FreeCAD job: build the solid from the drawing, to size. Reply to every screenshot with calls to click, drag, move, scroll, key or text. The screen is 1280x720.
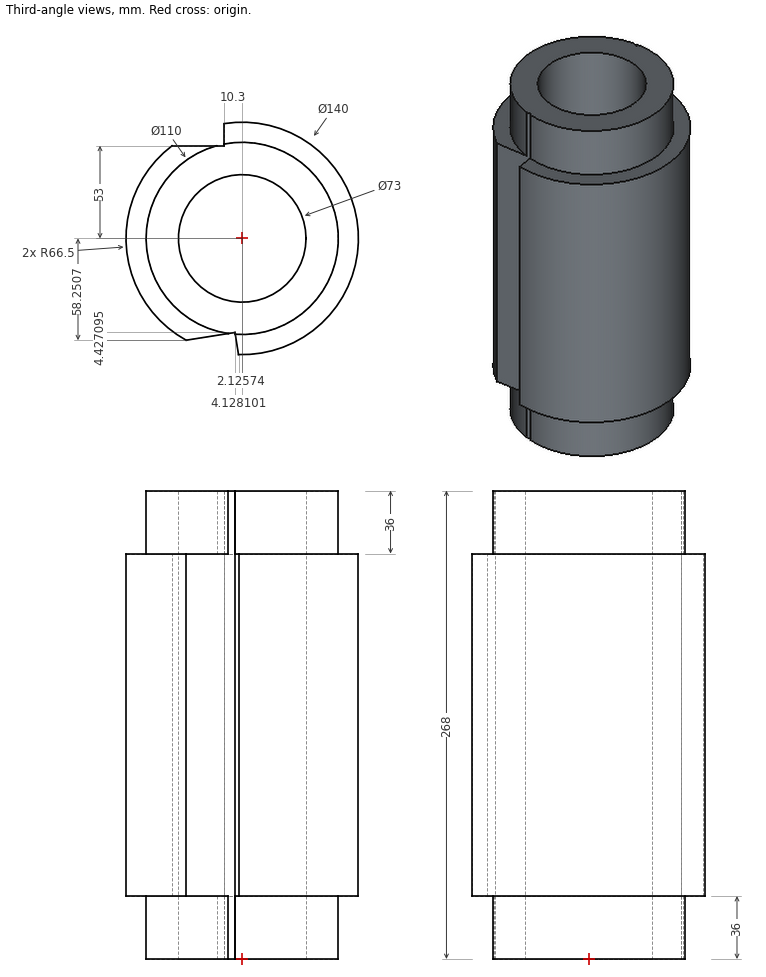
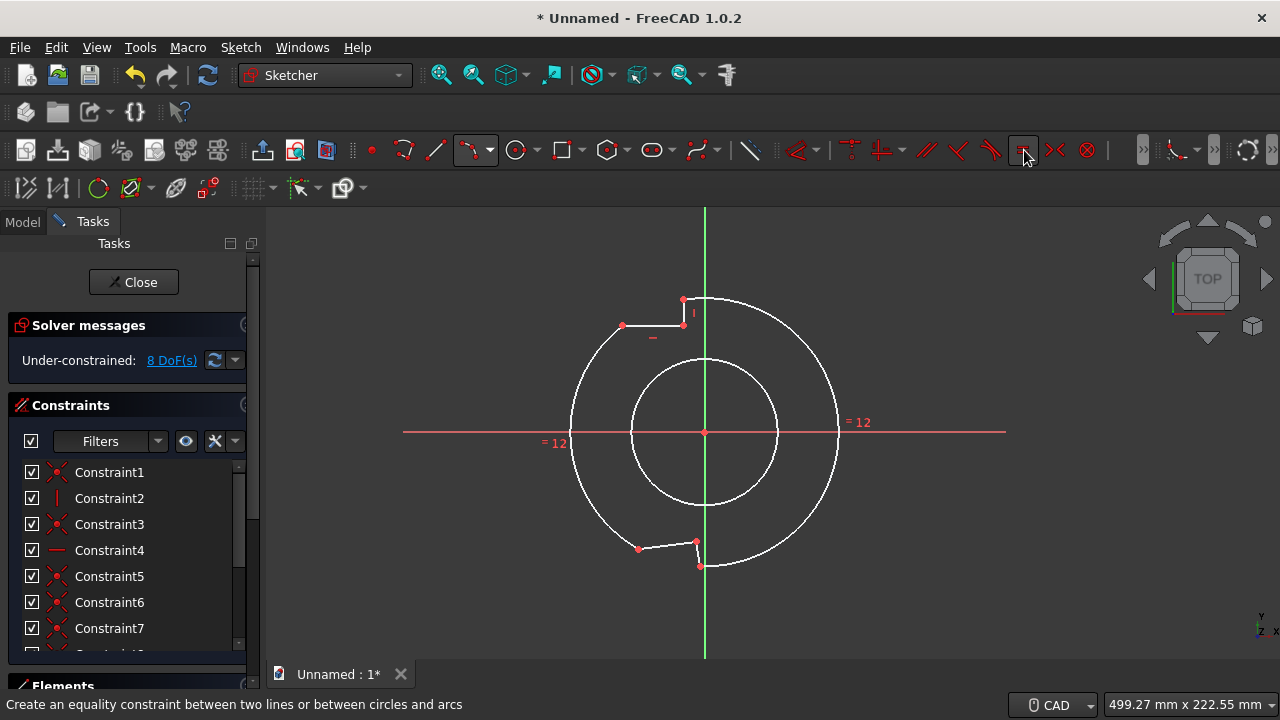
click(796, 150)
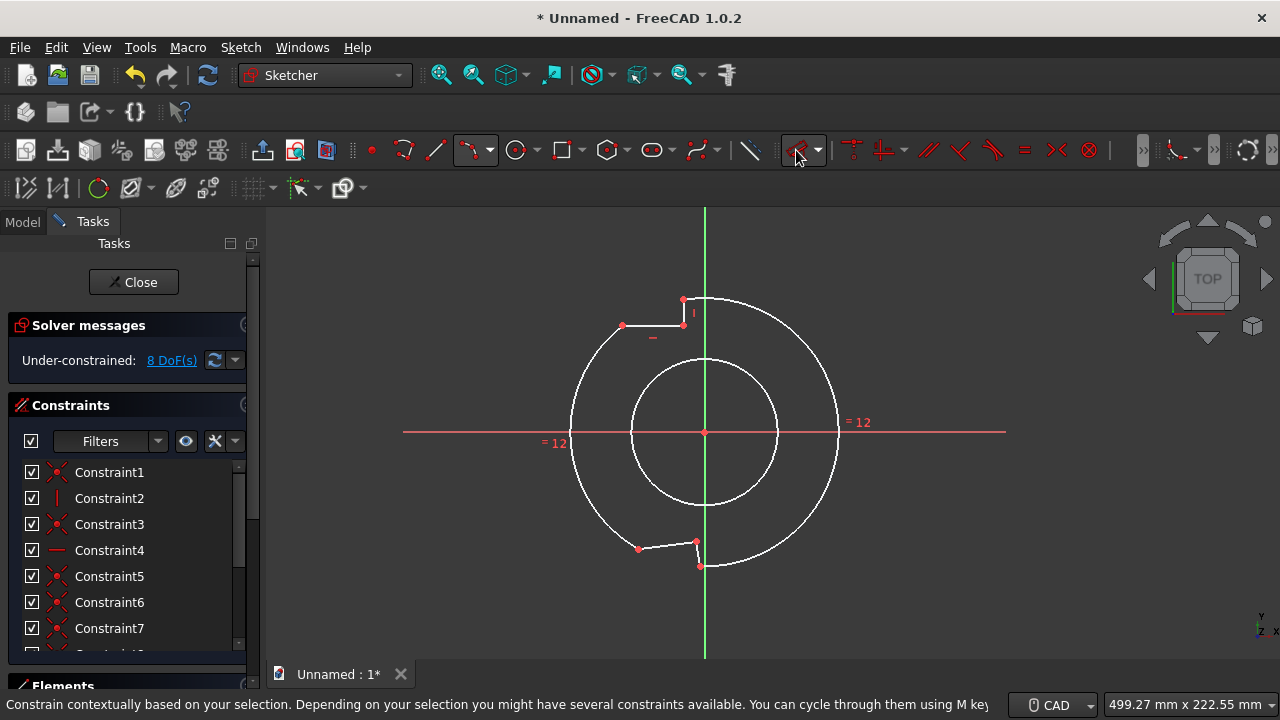
click(815, 508)
click(841, 526)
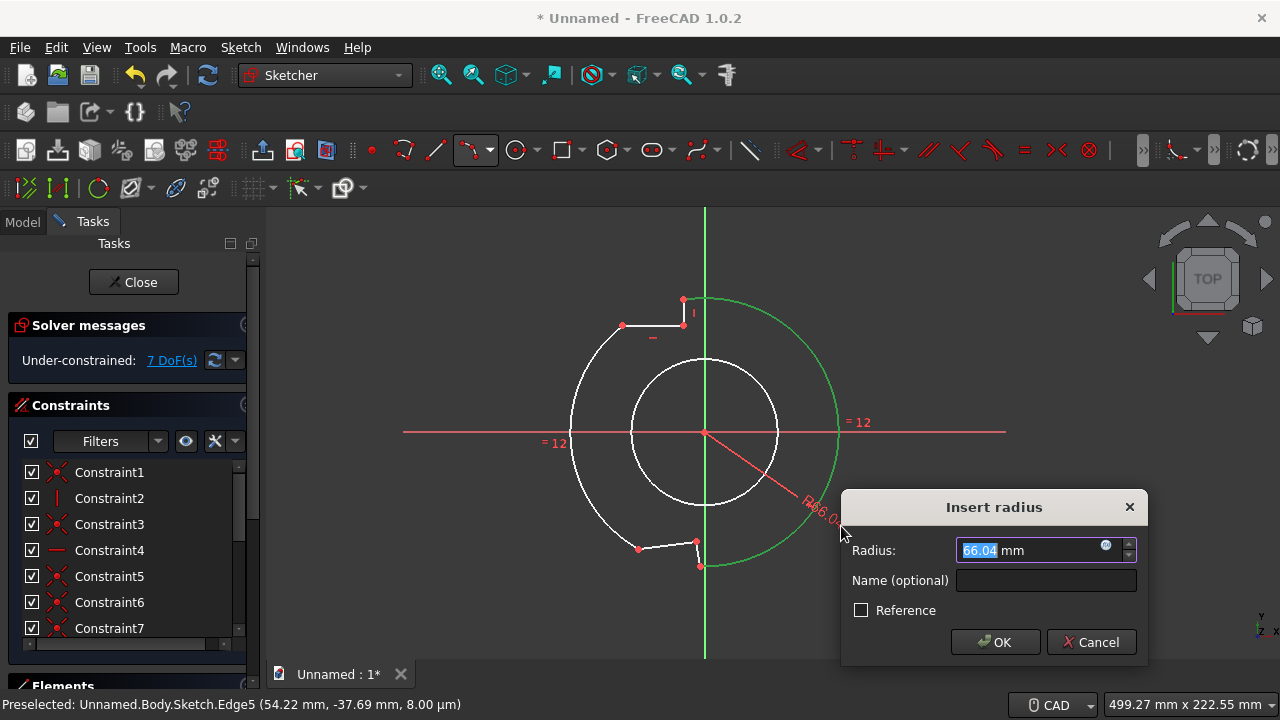
text(66.5)
key(Return)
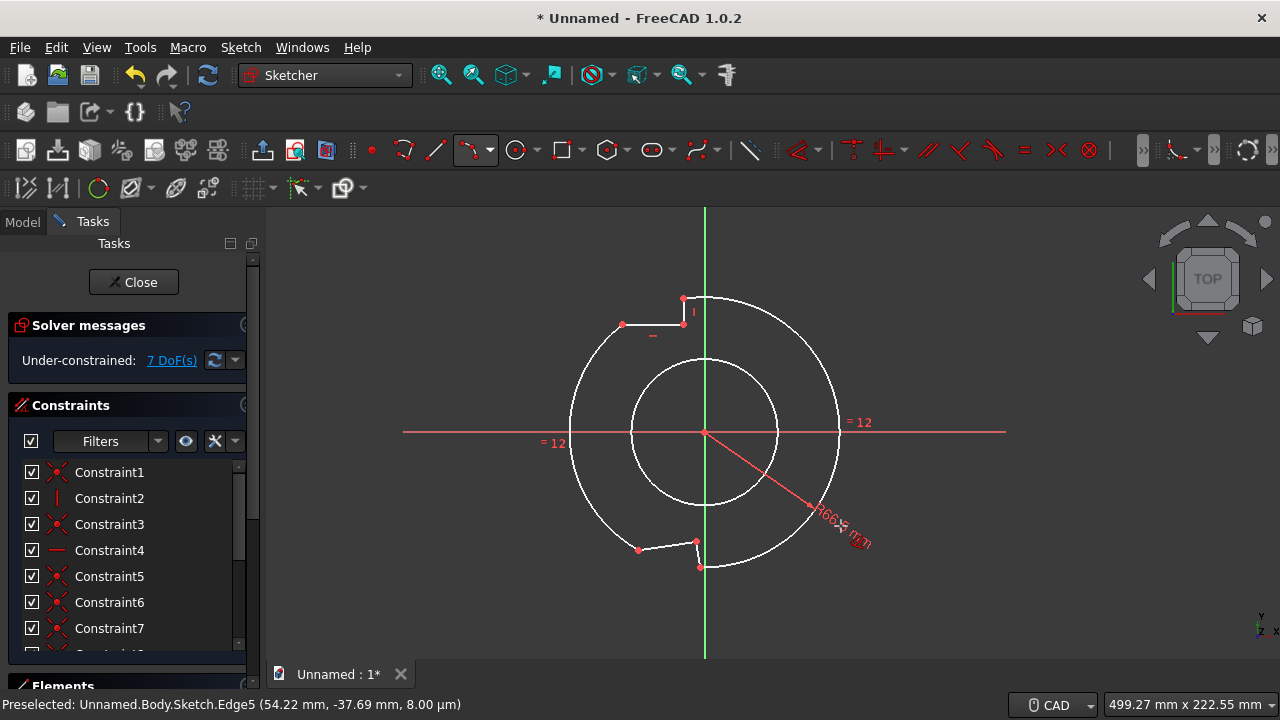
click(756, 380)
click(778, 357)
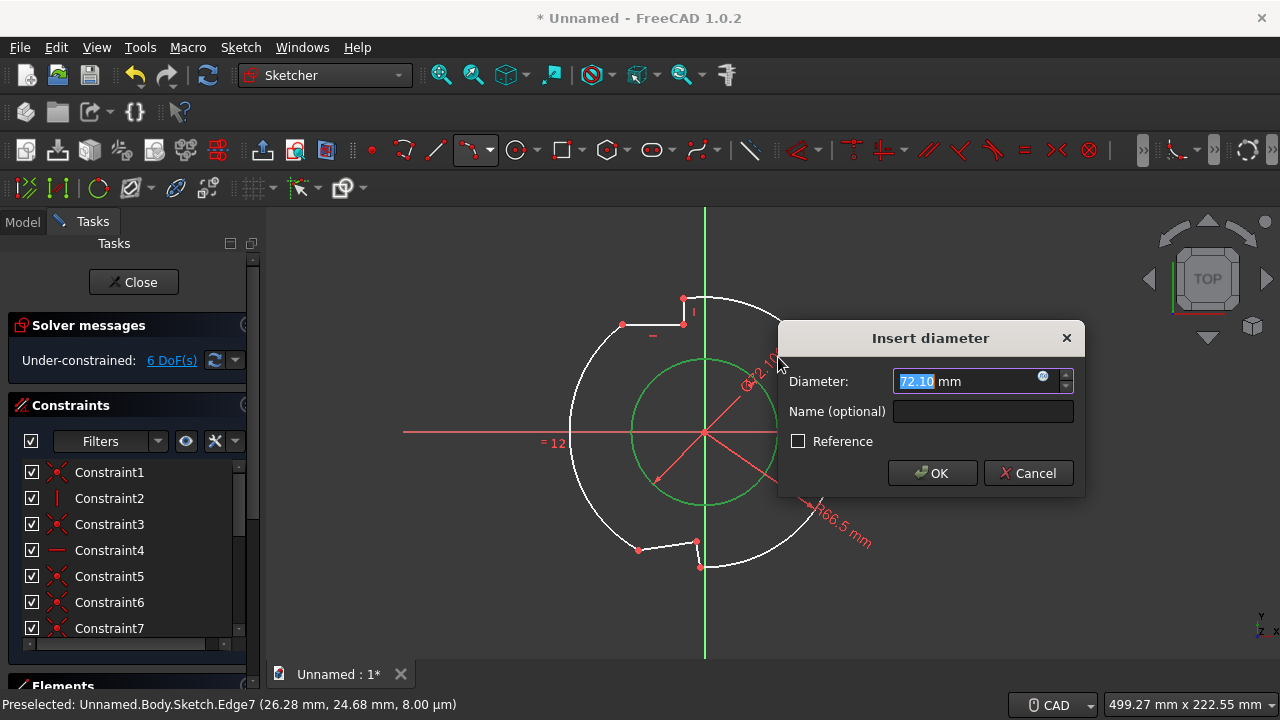
text(73)
key(Return)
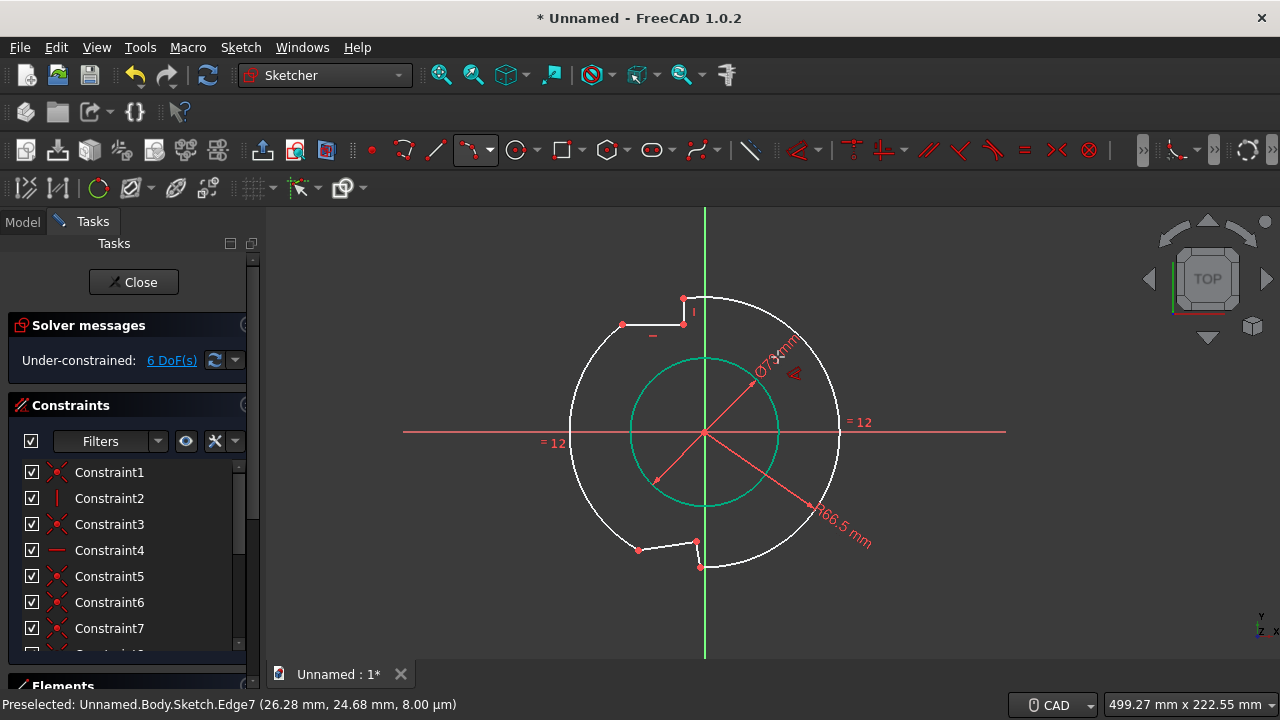
click(684, 325)
click(650, 354)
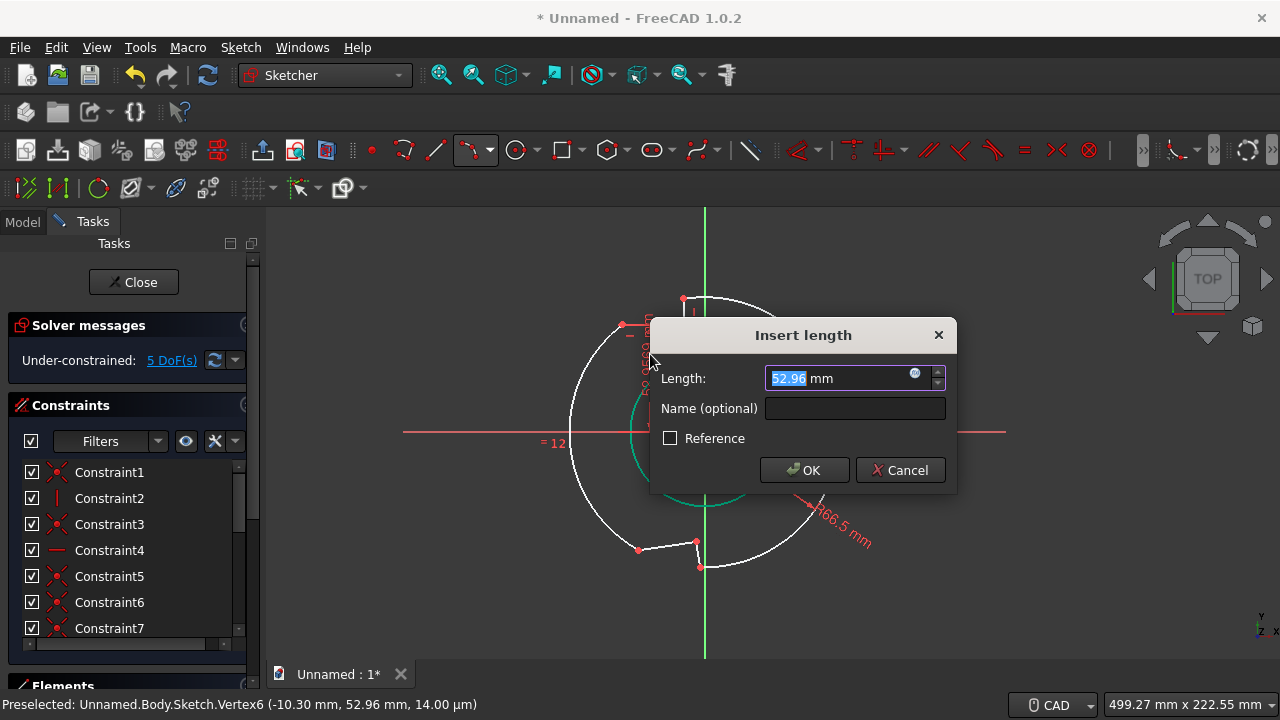
text(53)
key(Return)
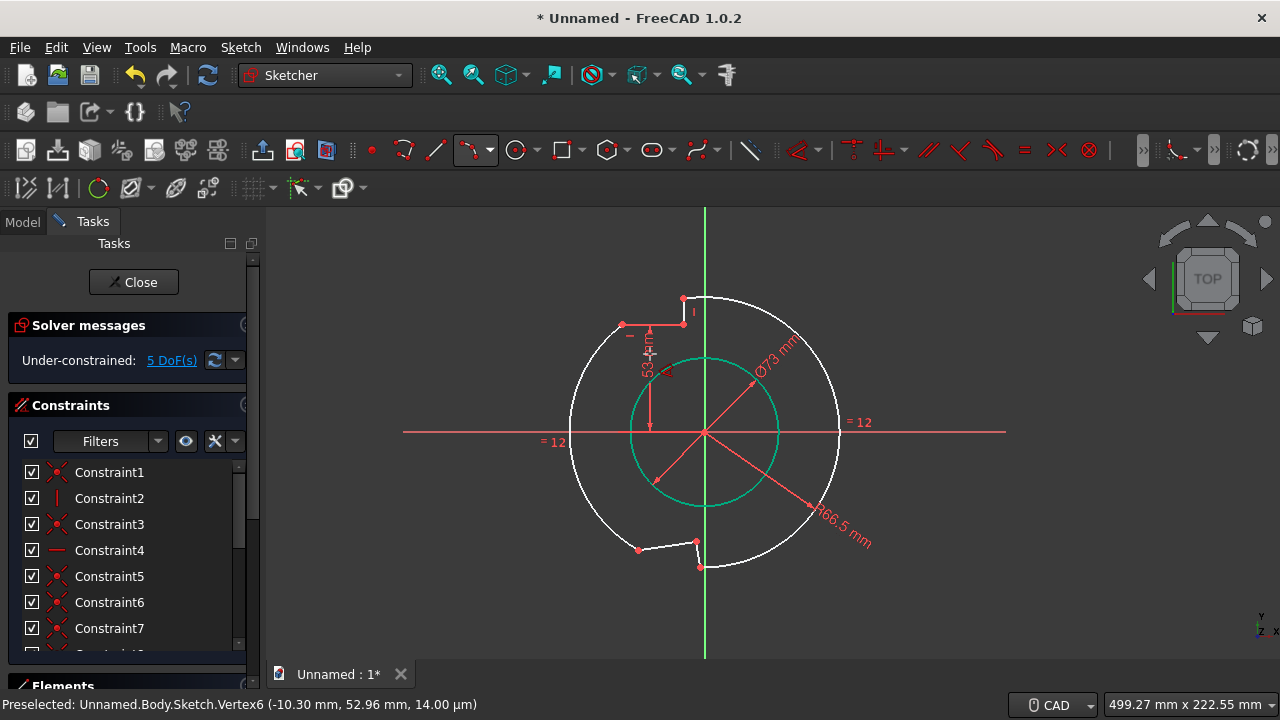
scroll(684, 299, up, 4)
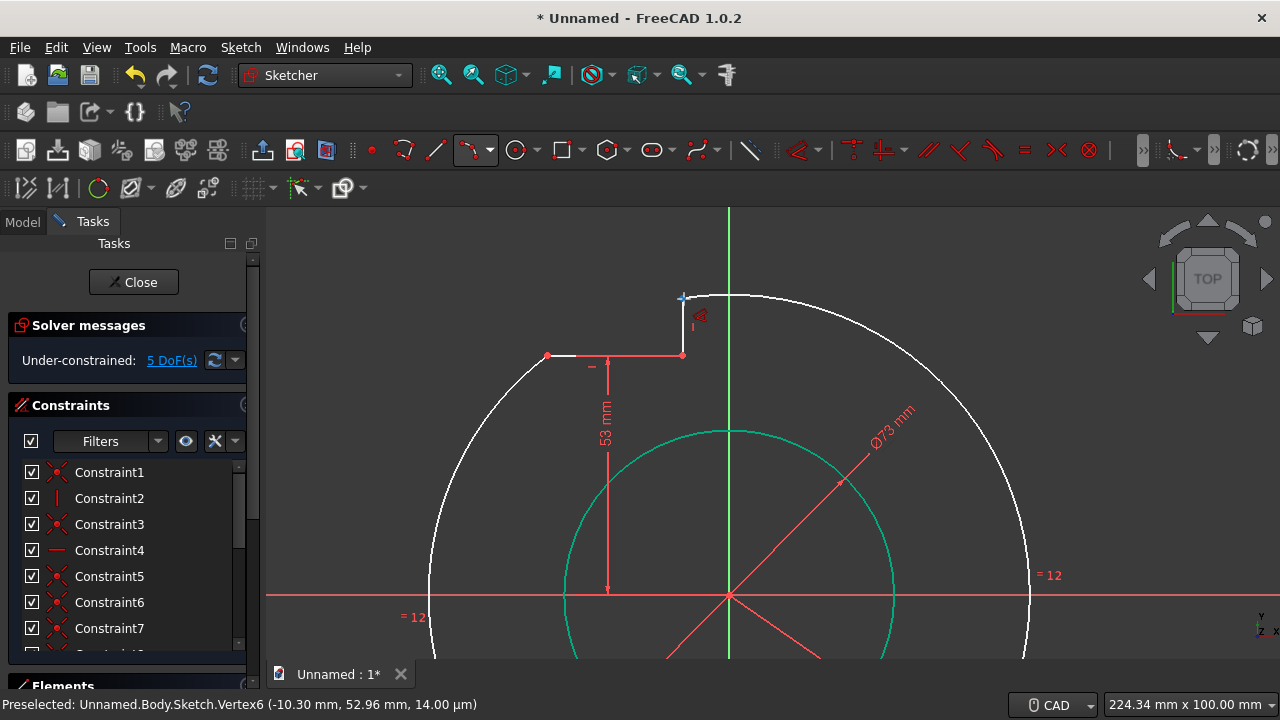
click(683, 298)
click(706, 264)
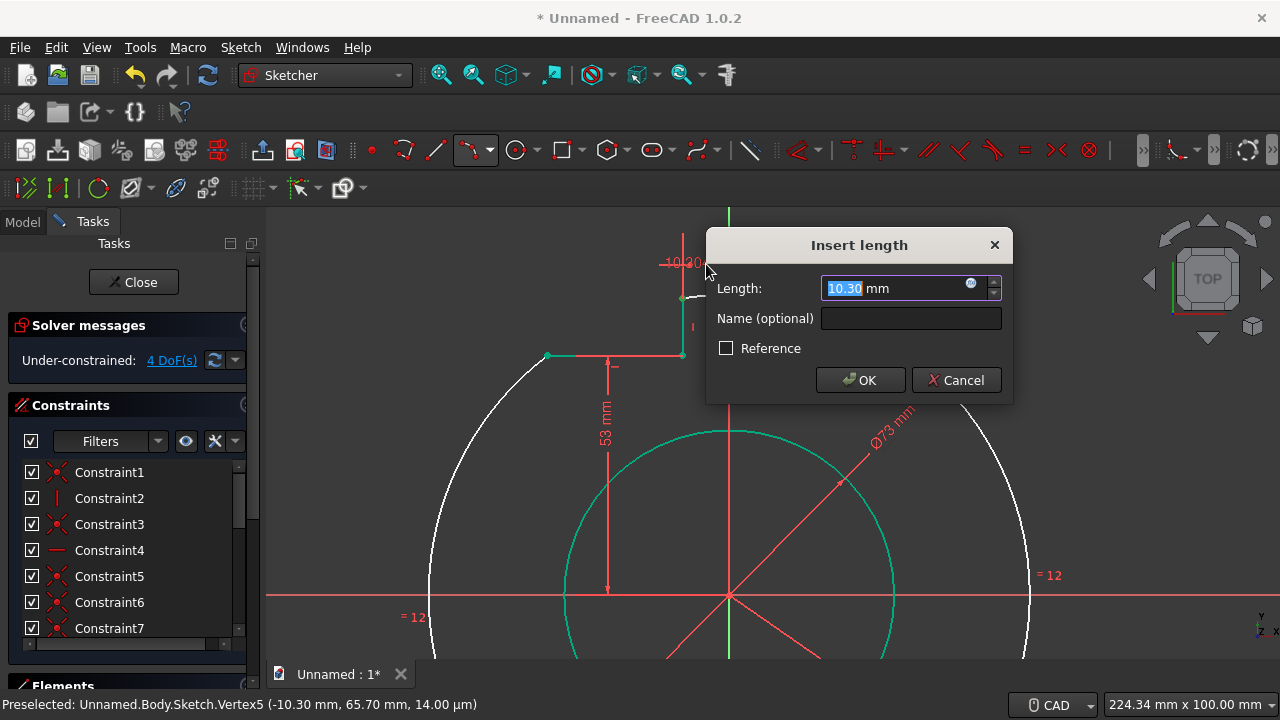
text(10.3)
key(Return)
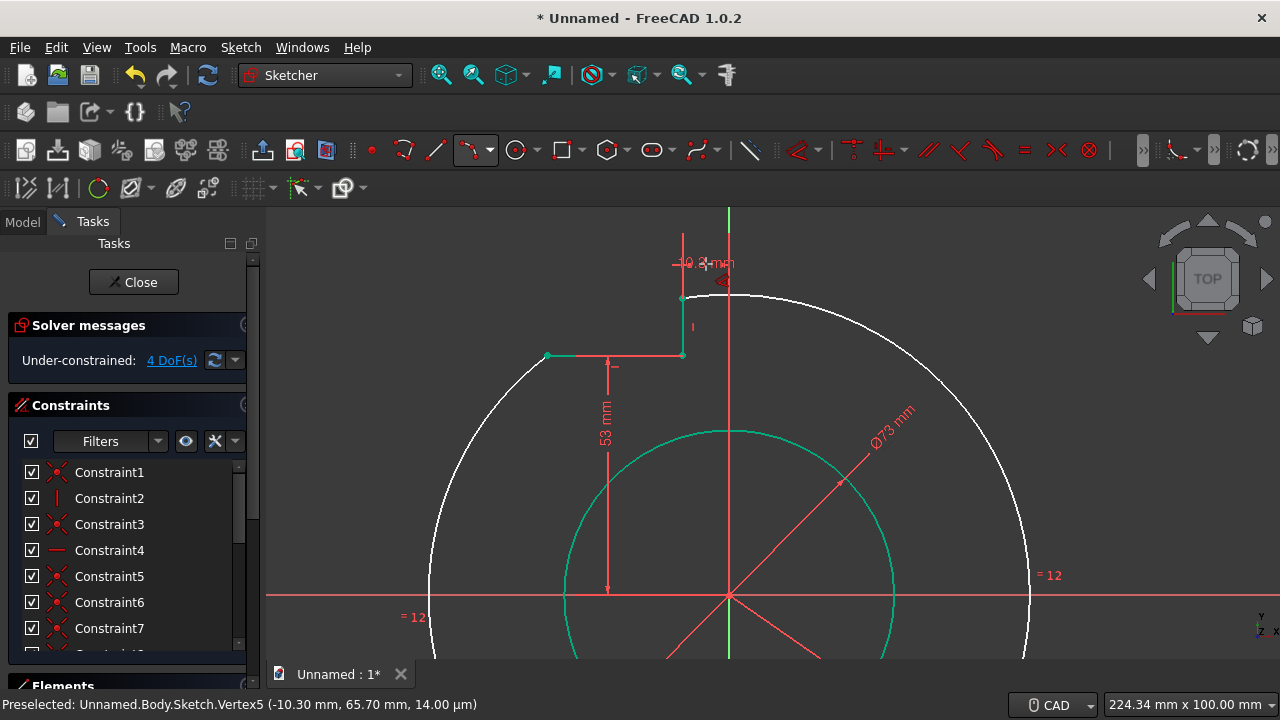
scroll(684, 299, down, 4)